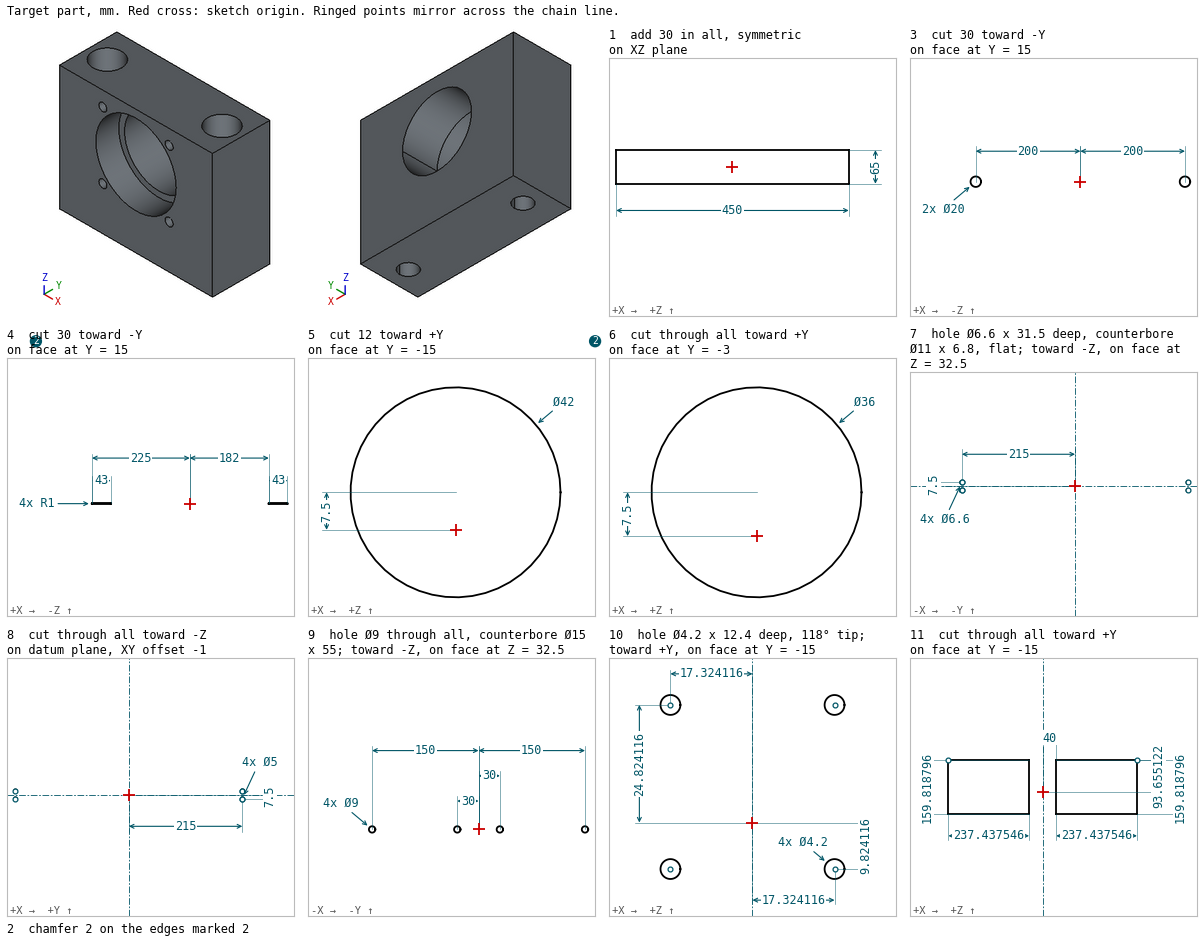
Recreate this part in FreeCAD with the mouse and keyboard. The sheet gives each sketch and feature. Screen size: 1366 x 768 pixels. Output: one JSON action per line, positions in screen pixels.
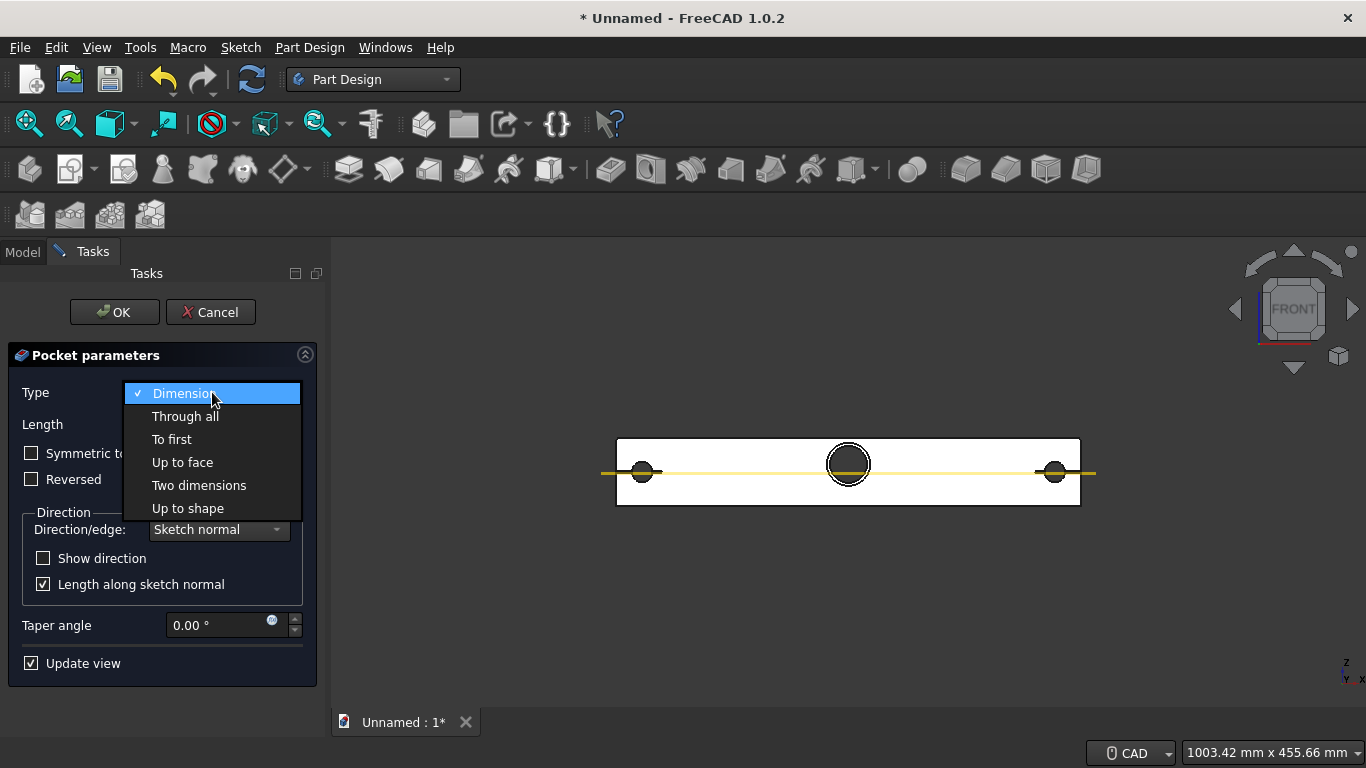
{"action": "left_click", "coordinate": [212, 416]}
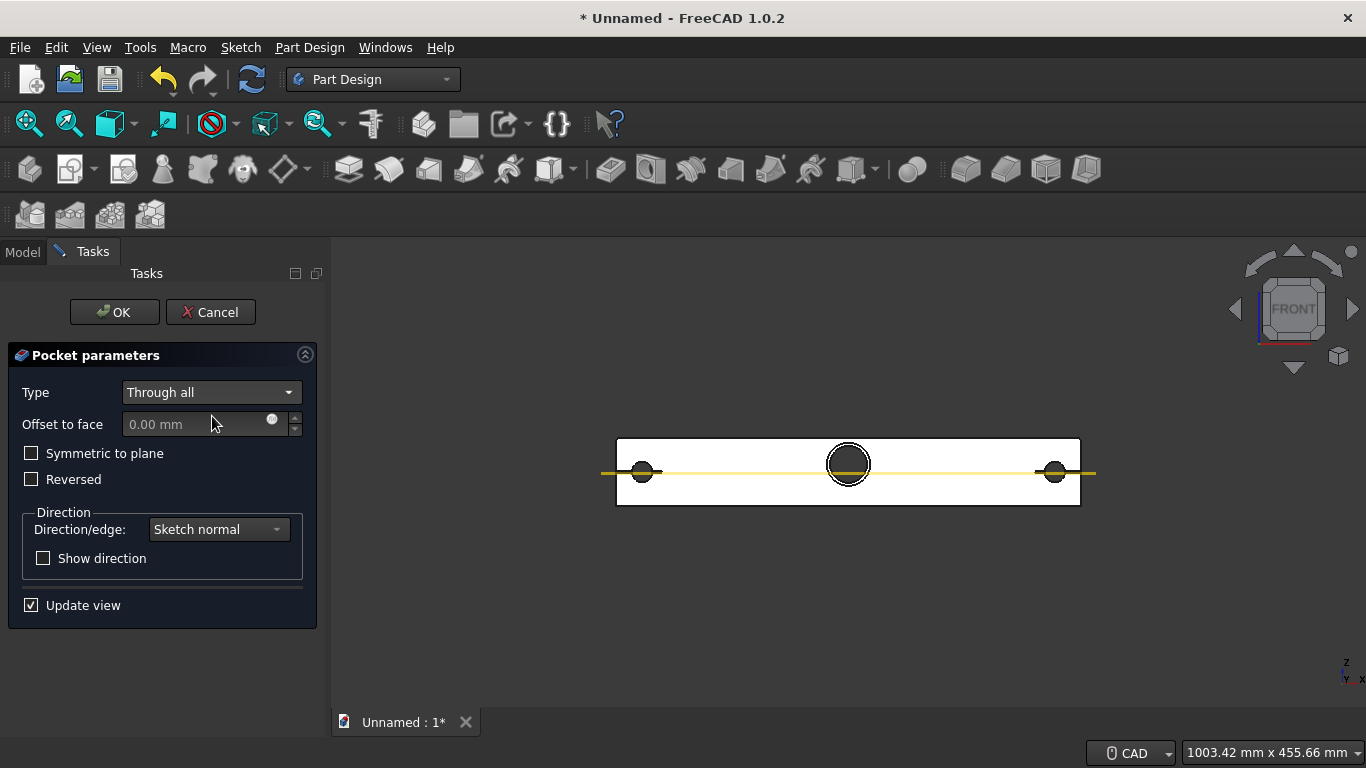
{"action": "left_click", "coordinate": [115, 312]}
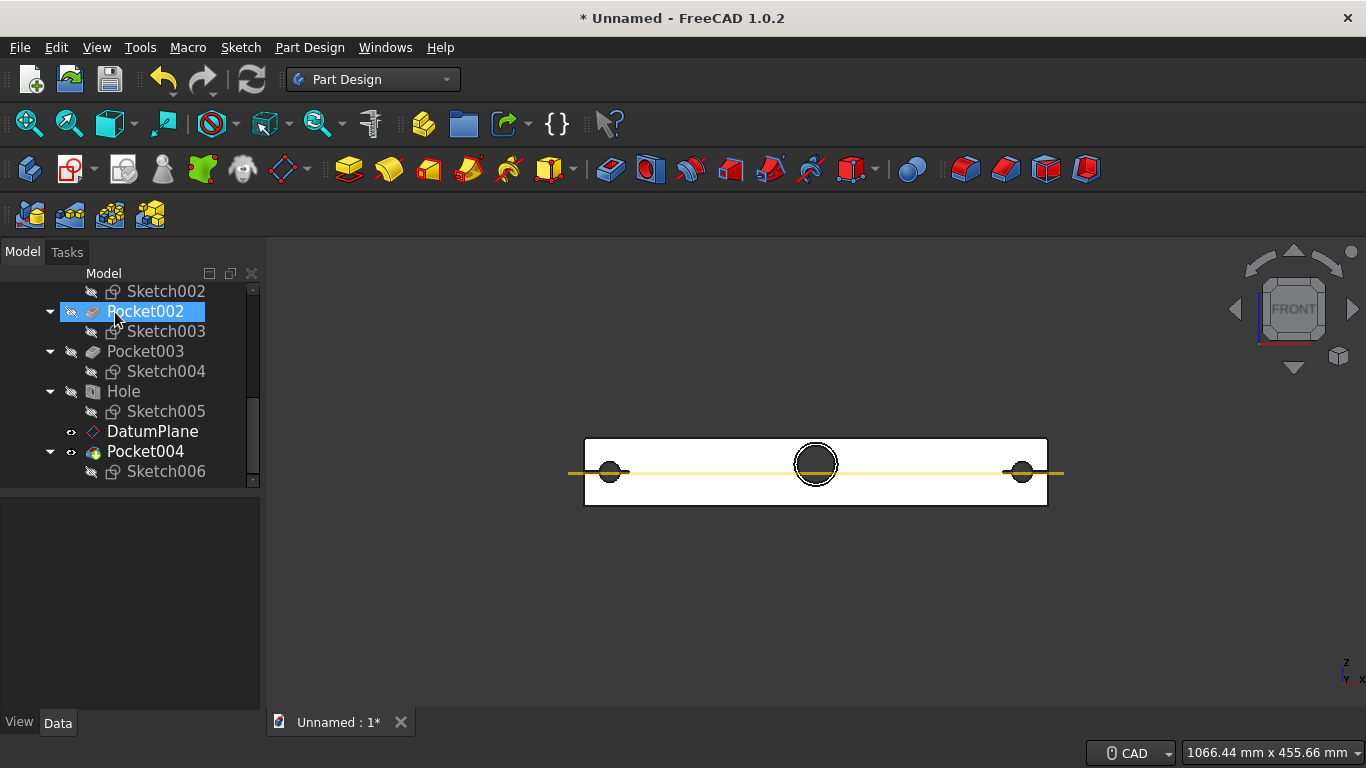
{"action": "left_click", "coordinate": [116, 432]}
{"action": "key", "text": "space"}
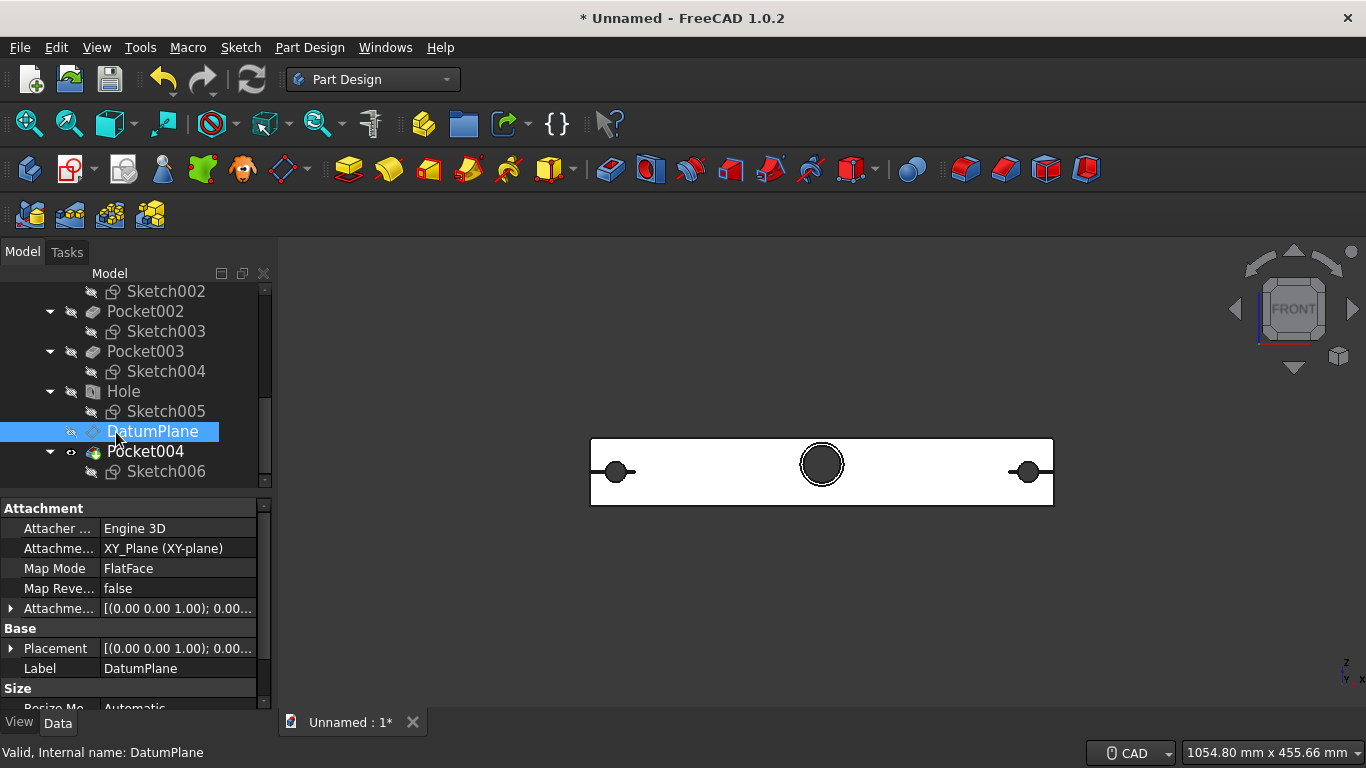
{"action": "key", "text": "v f"}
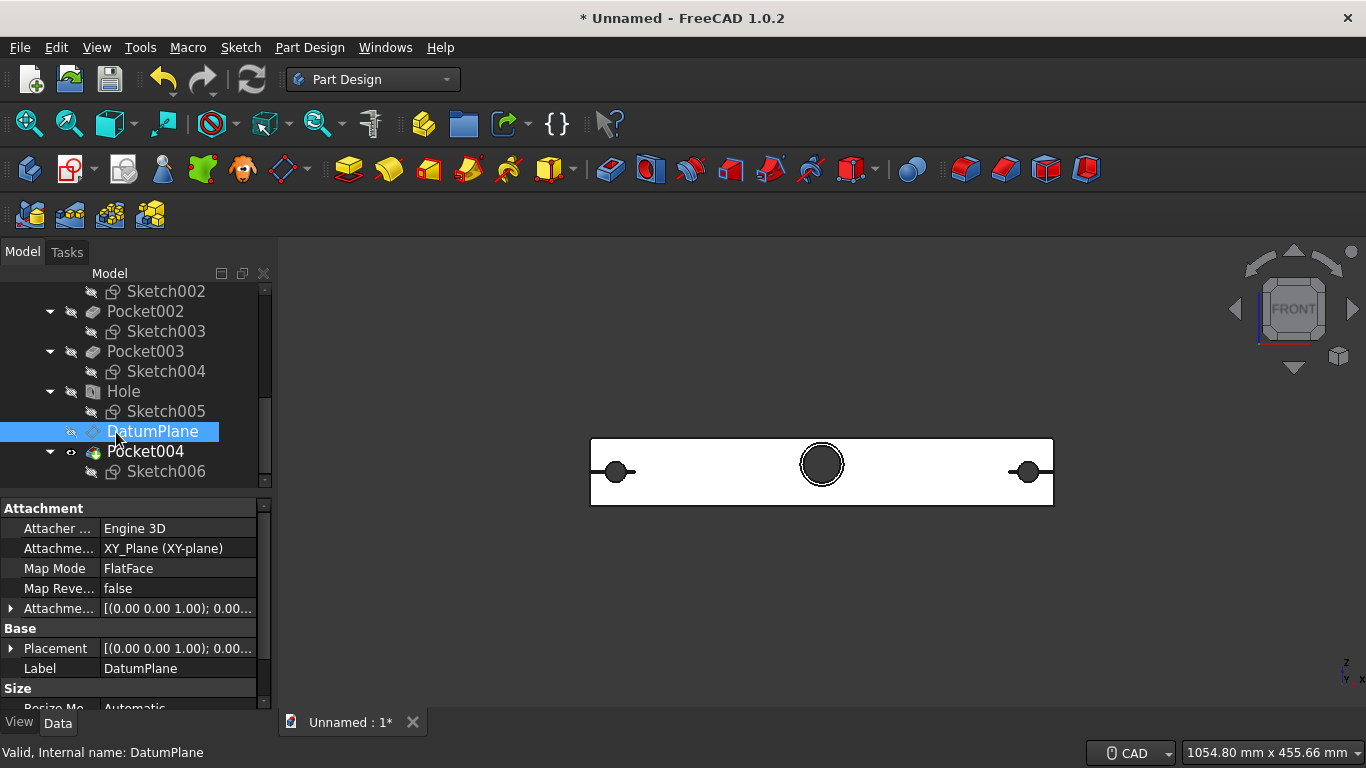
{"action": "key", "text": "0"}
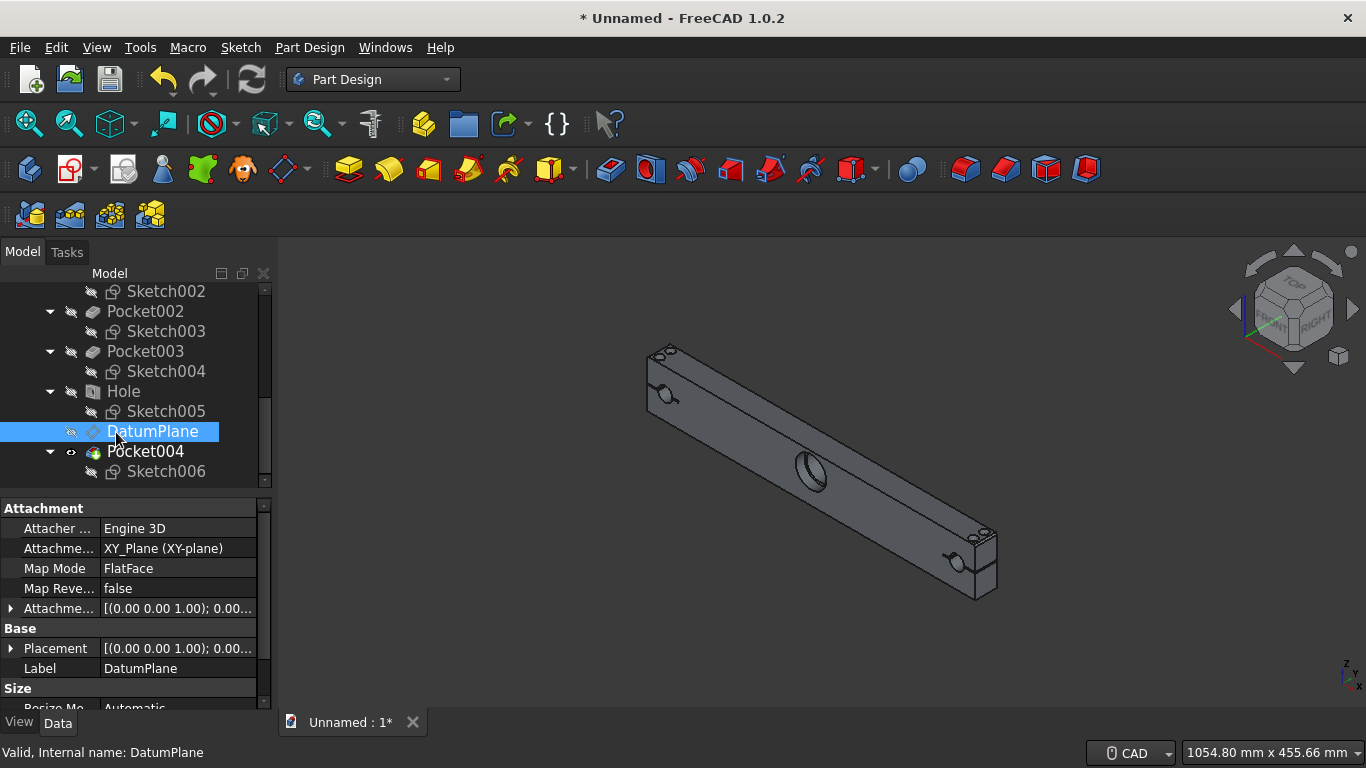
{"action": "left_click", "coordinate": [961, 524]}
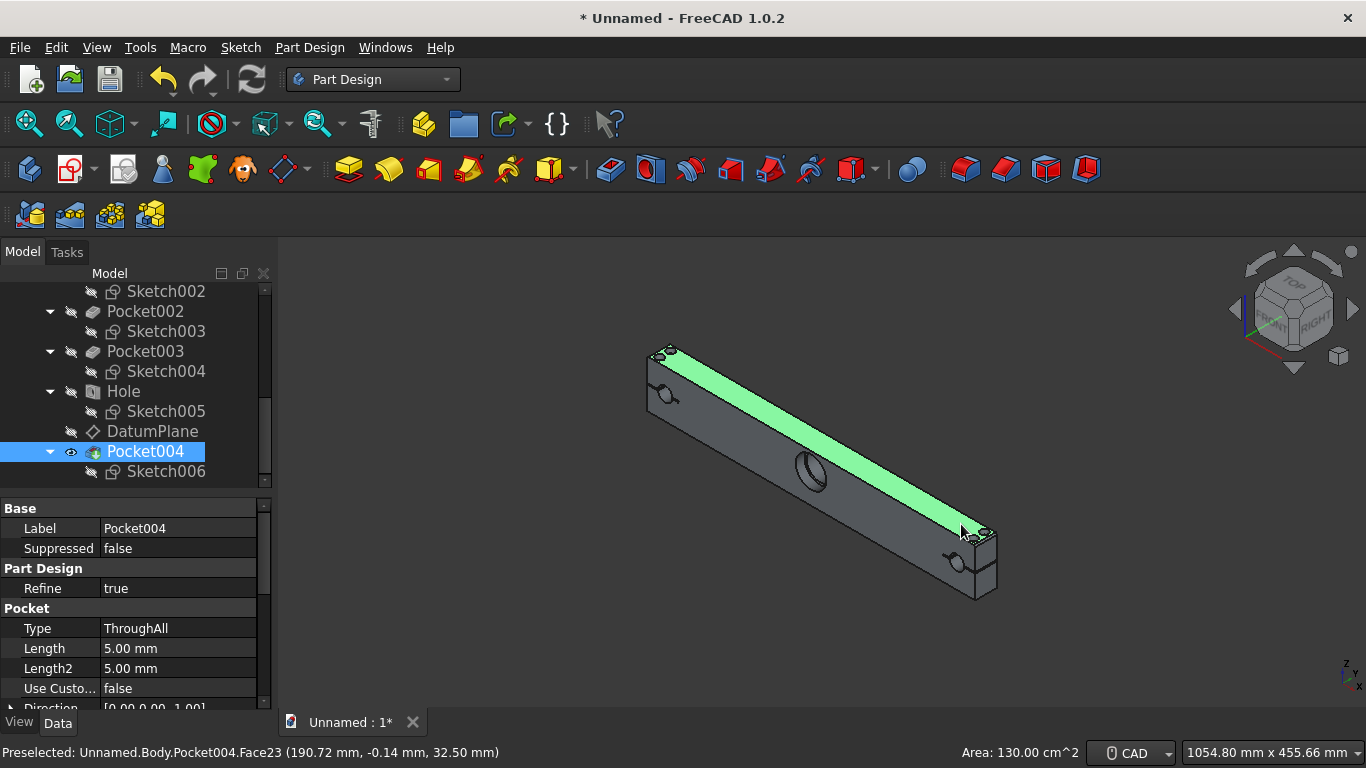
{"action": "left_click", "coordinate": [70, 170]}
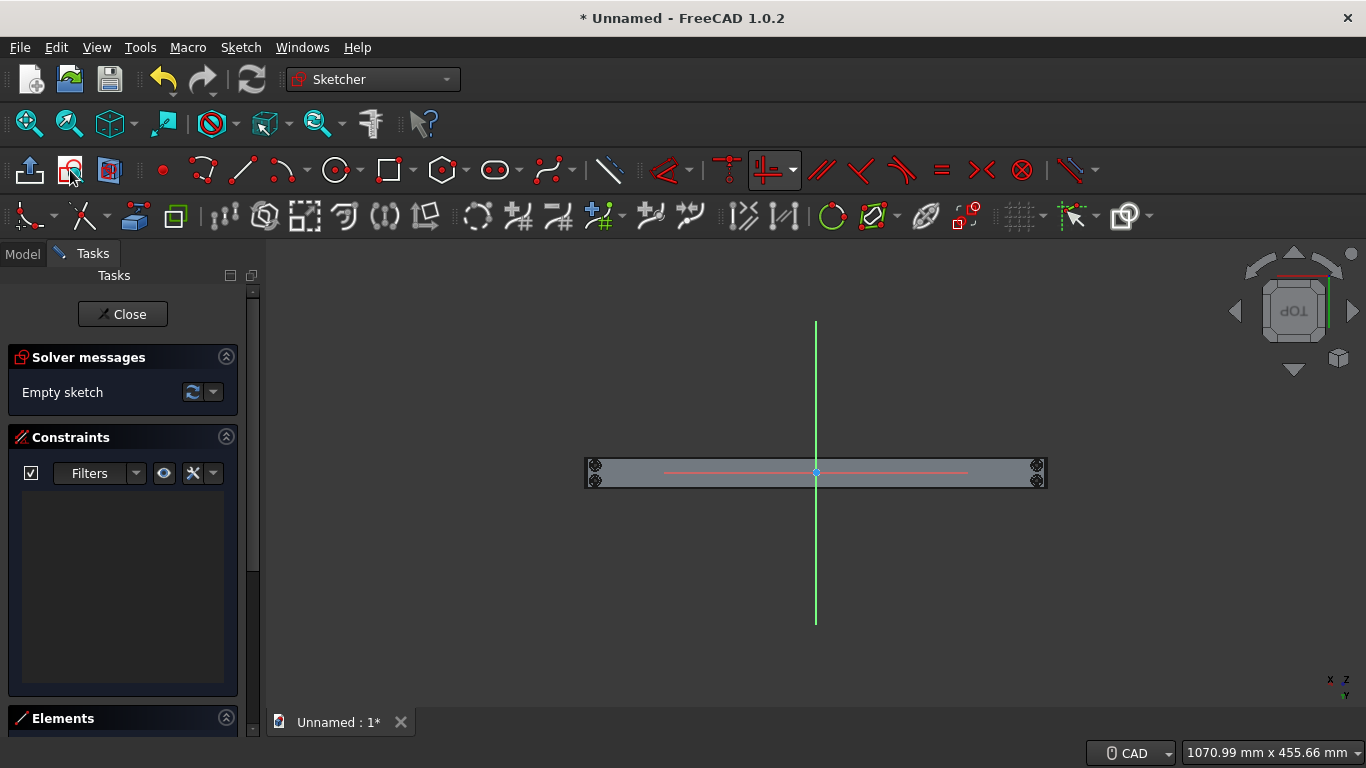
{"action": "scroll", "coordinate": [872, 473], "scroll_direction": "up", "scroll_amount": 4}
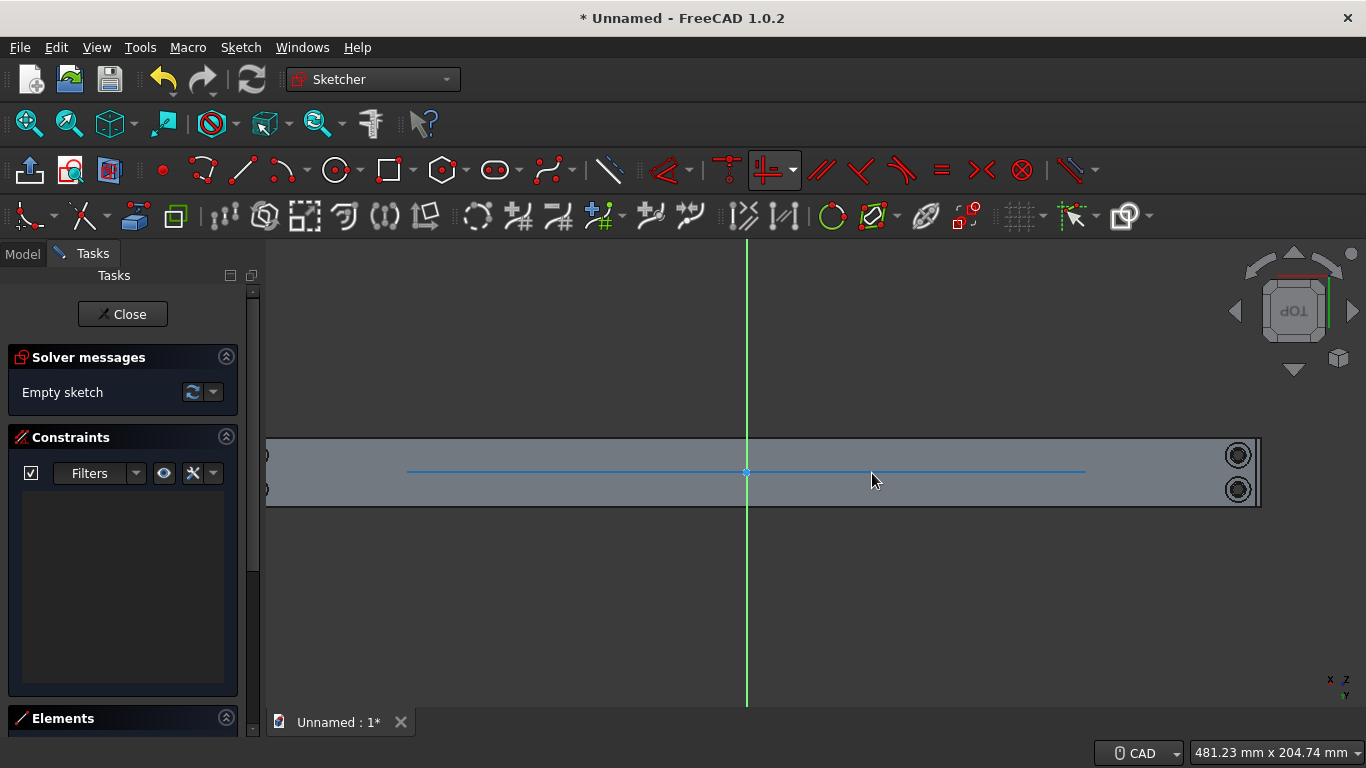
{"action": "left_click", "coordinate": [336, 170]}